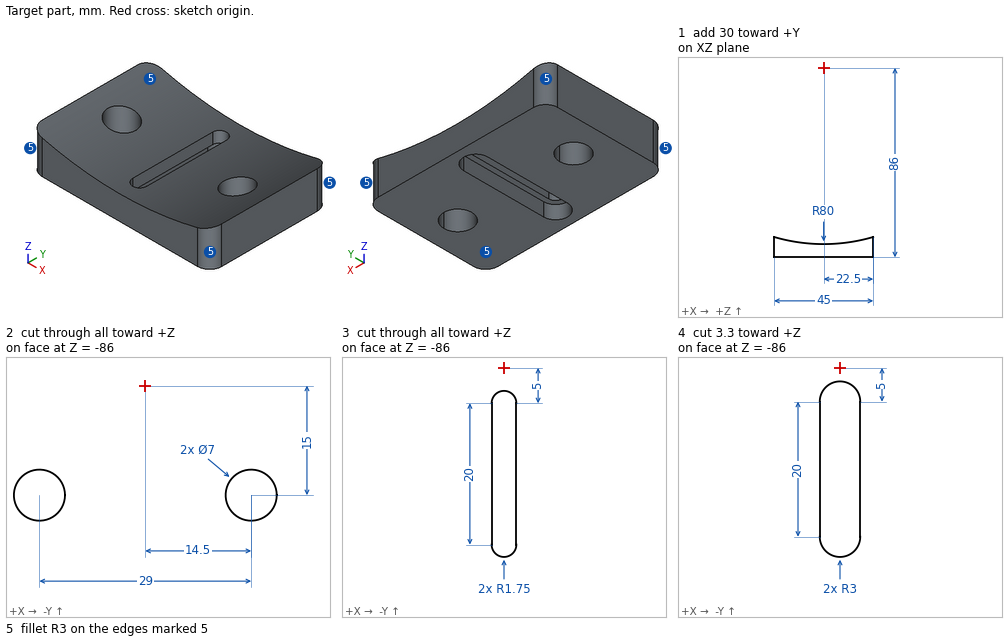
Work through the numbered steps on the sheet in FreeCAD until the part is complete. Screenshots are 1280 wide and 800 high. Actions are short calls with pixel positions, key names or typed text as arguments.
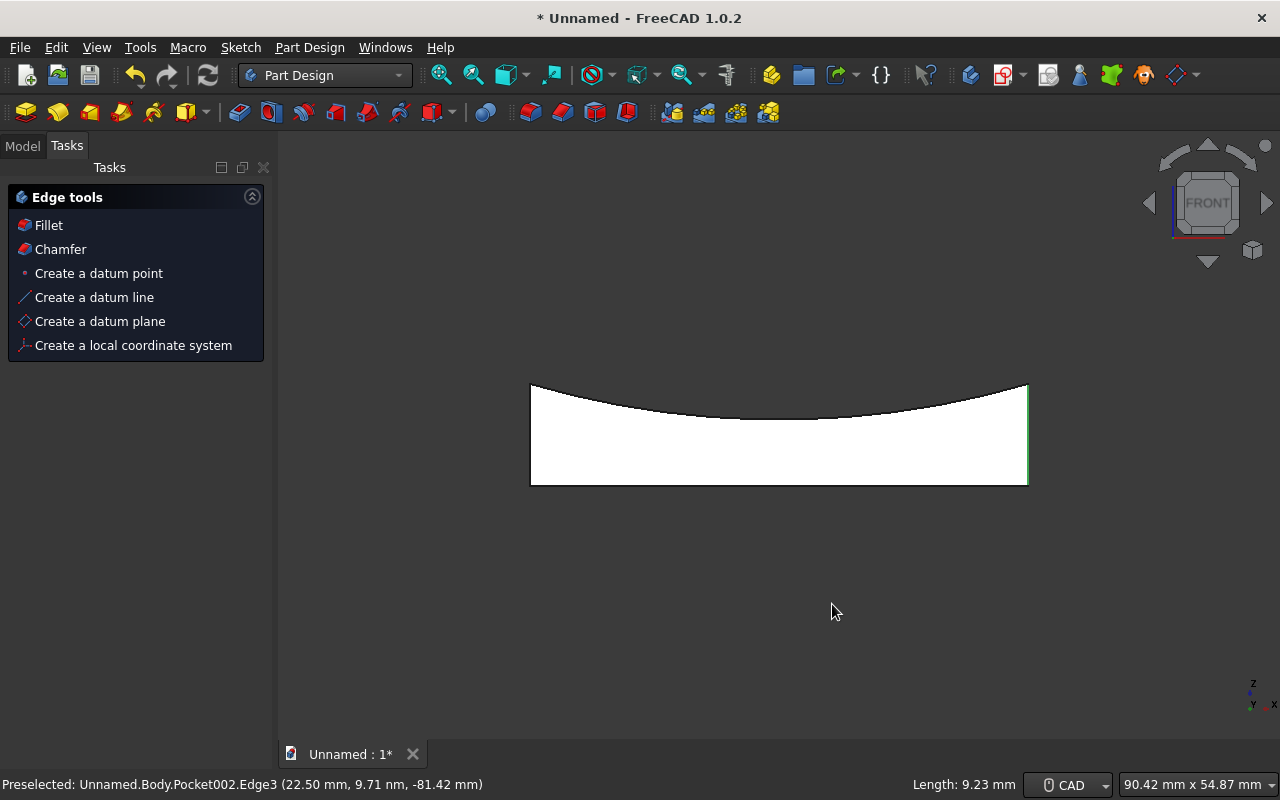
click(530, 473, ctrl)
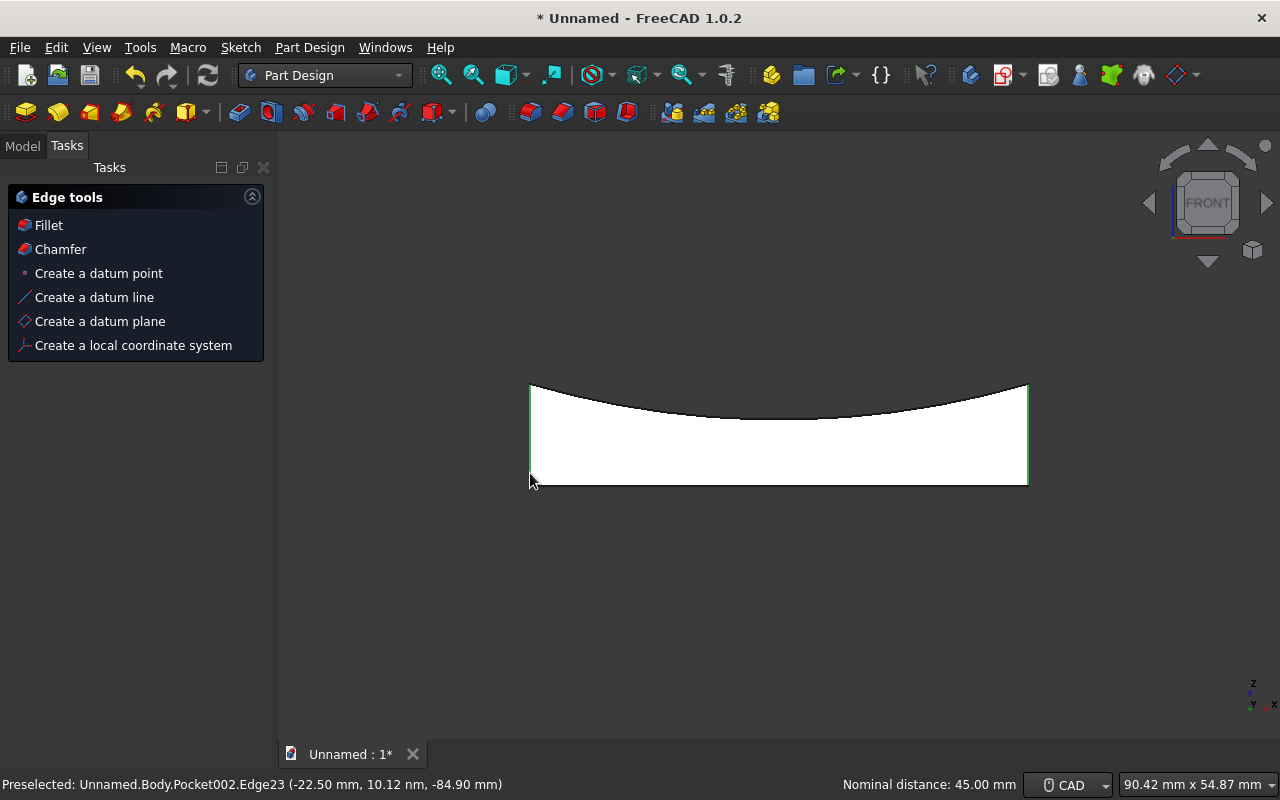
key(3)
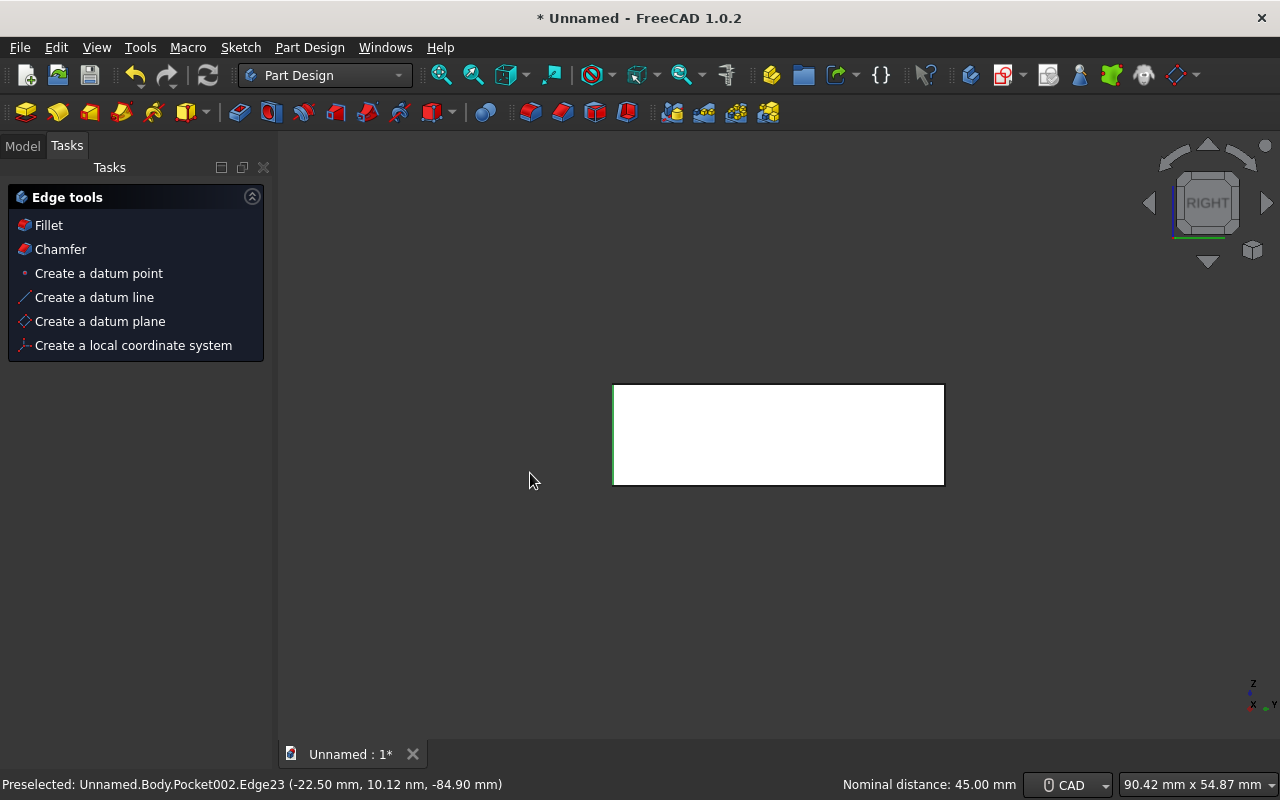
key(v)
key(f)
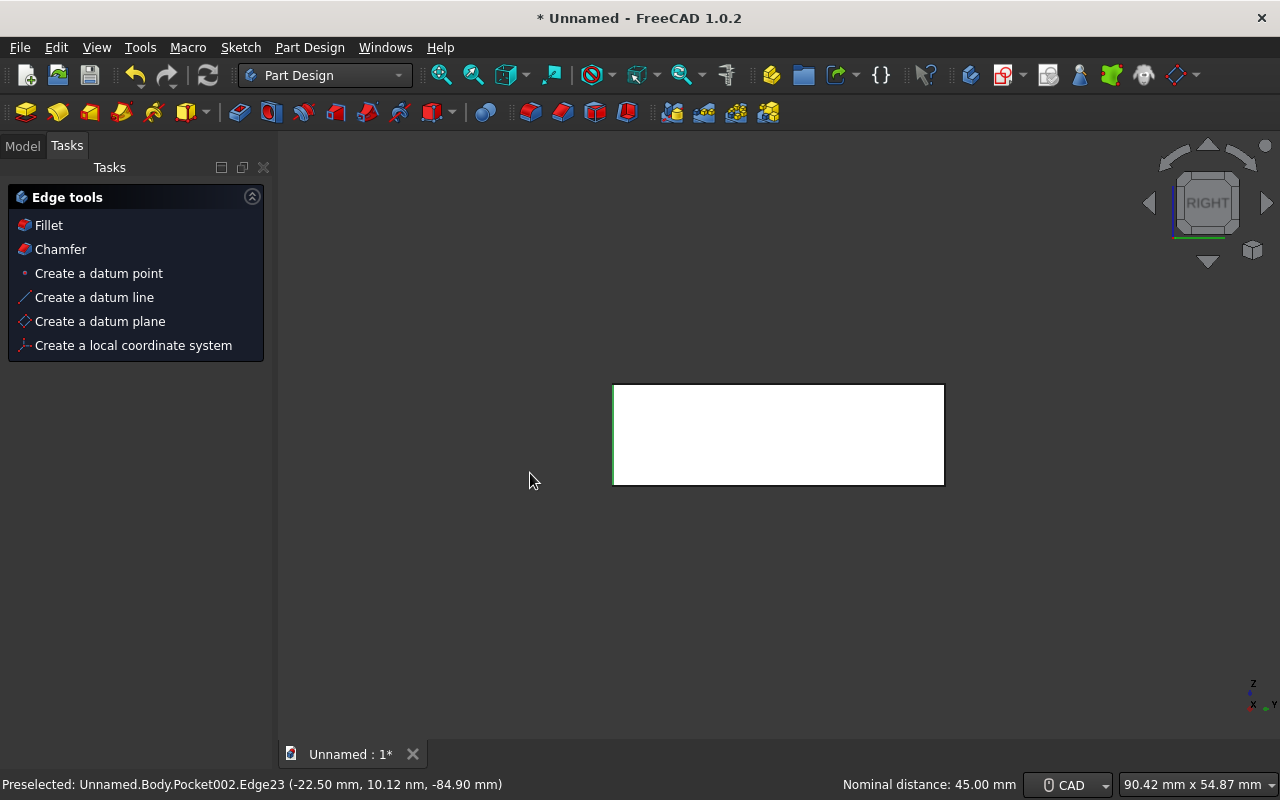
click(945, 434, ctrl)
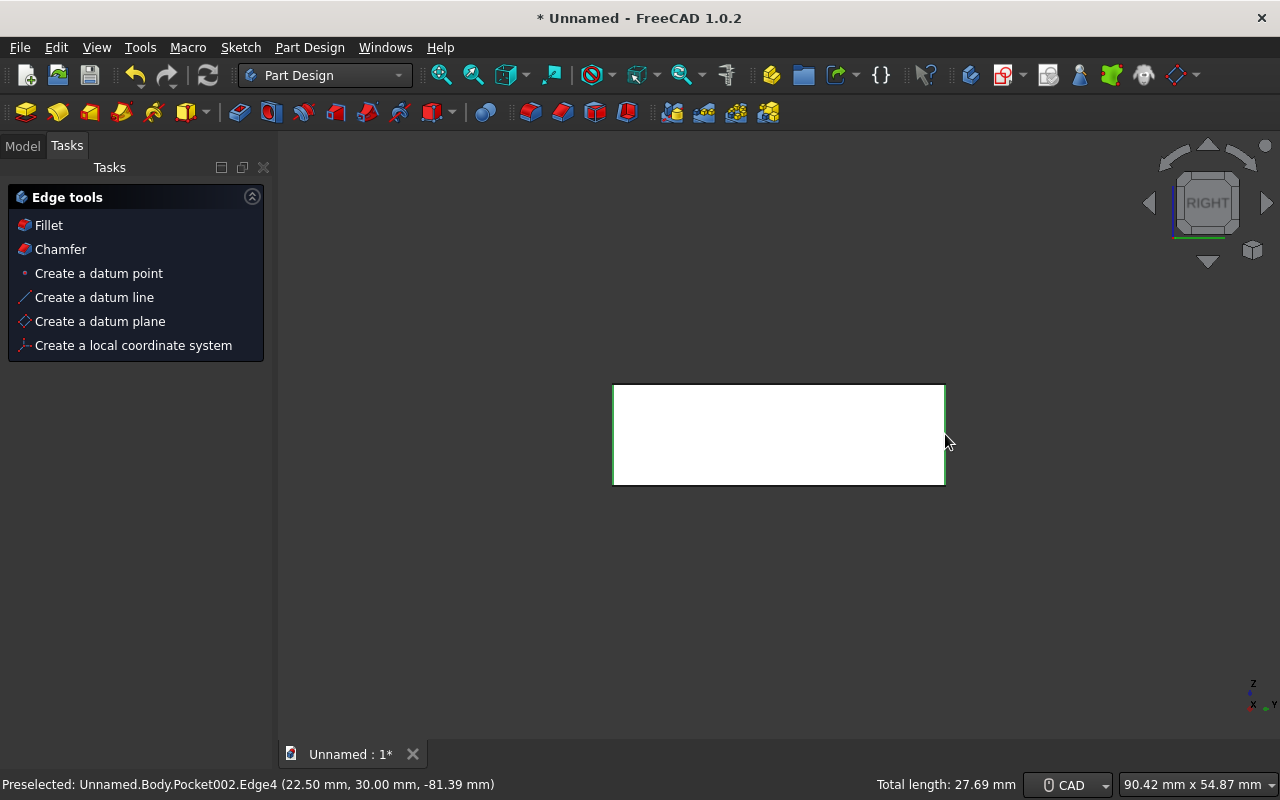
key(5)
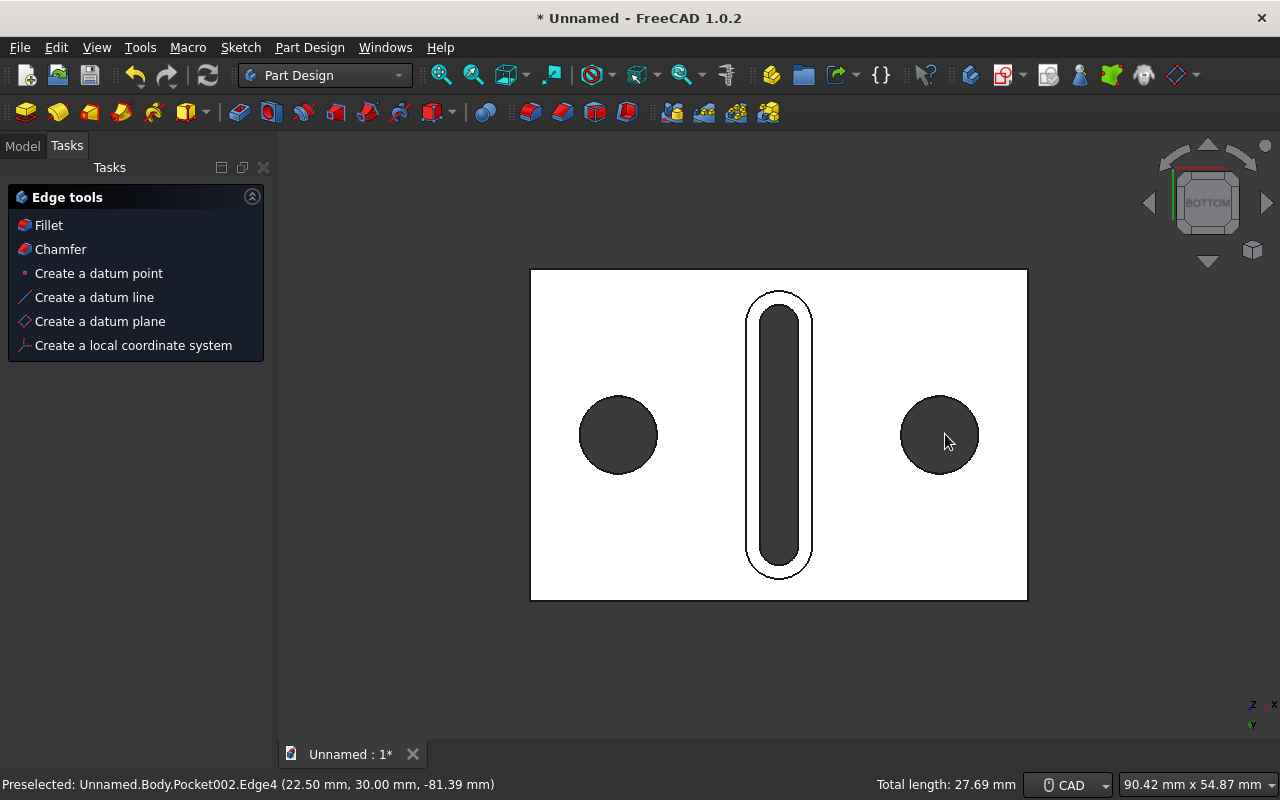
key(4)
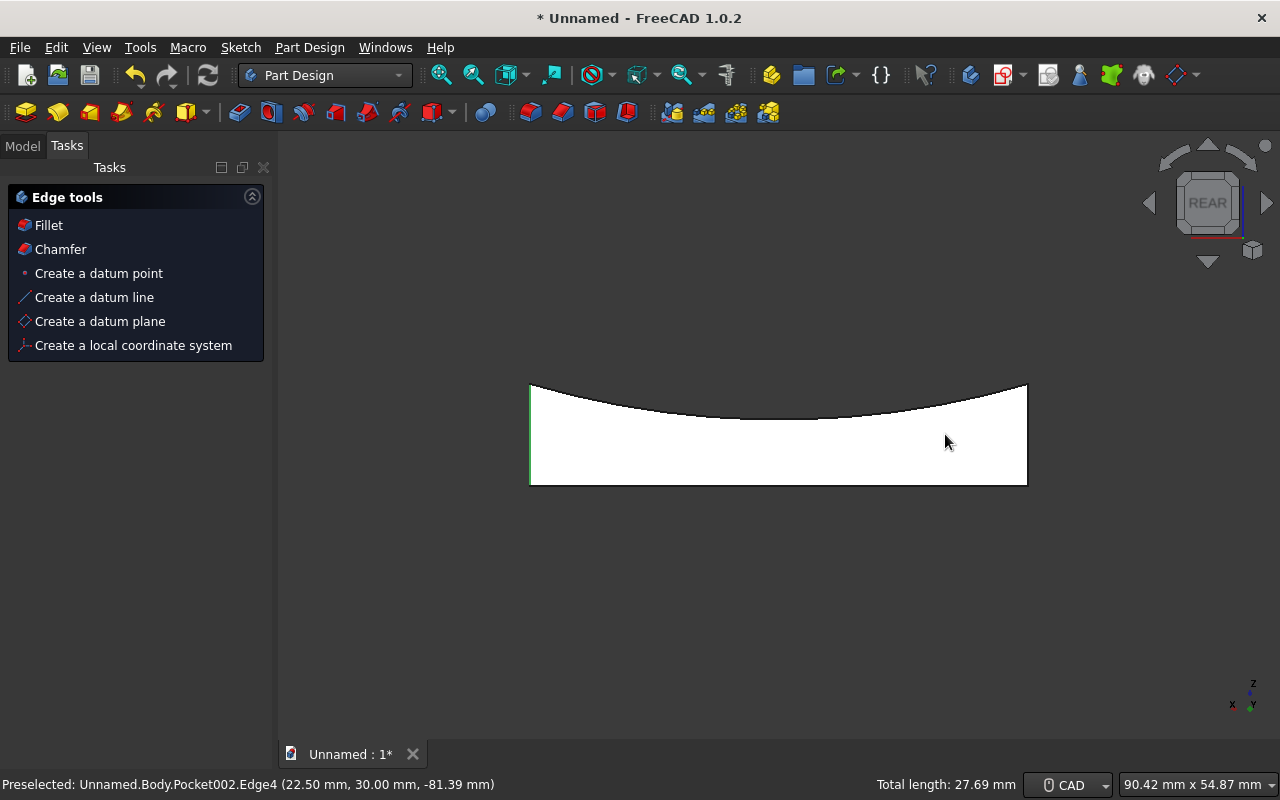
click(1028, 434, ctrl)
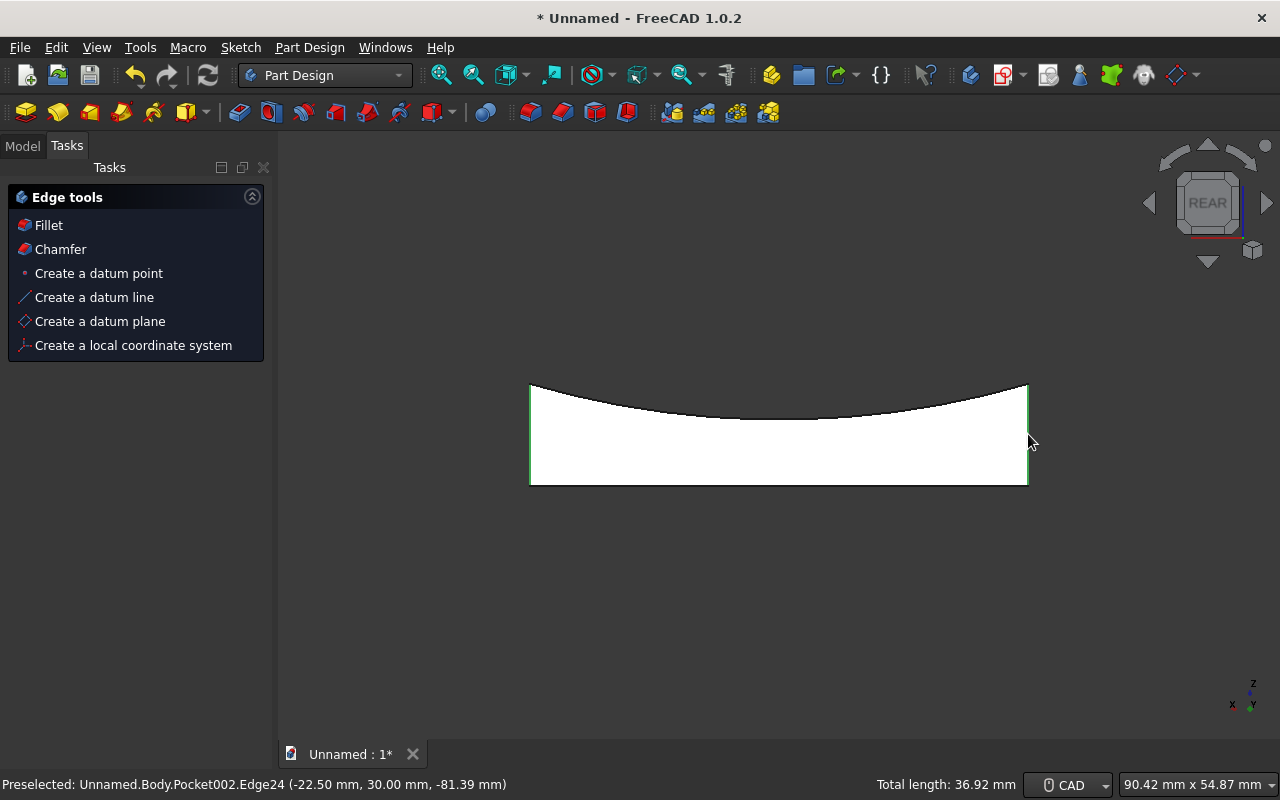
click(532, 112)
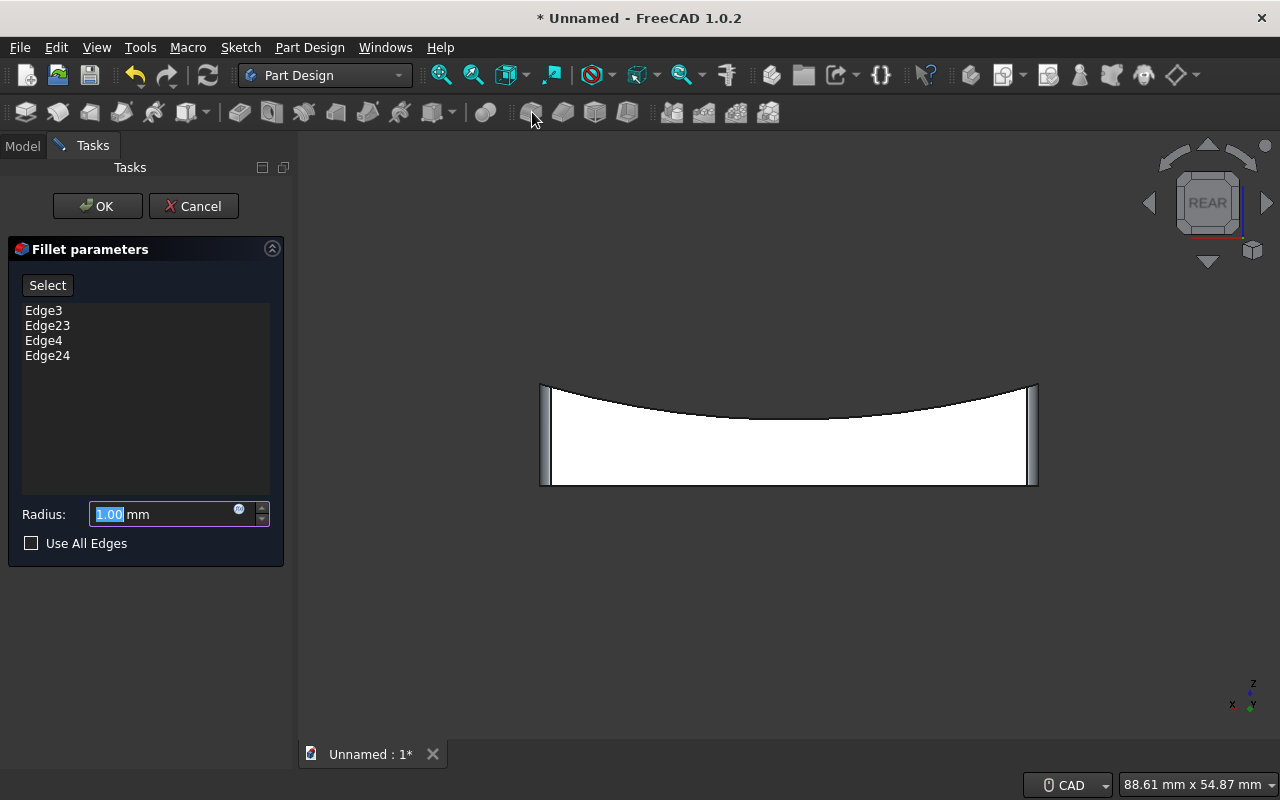
text(3)
key(Tab)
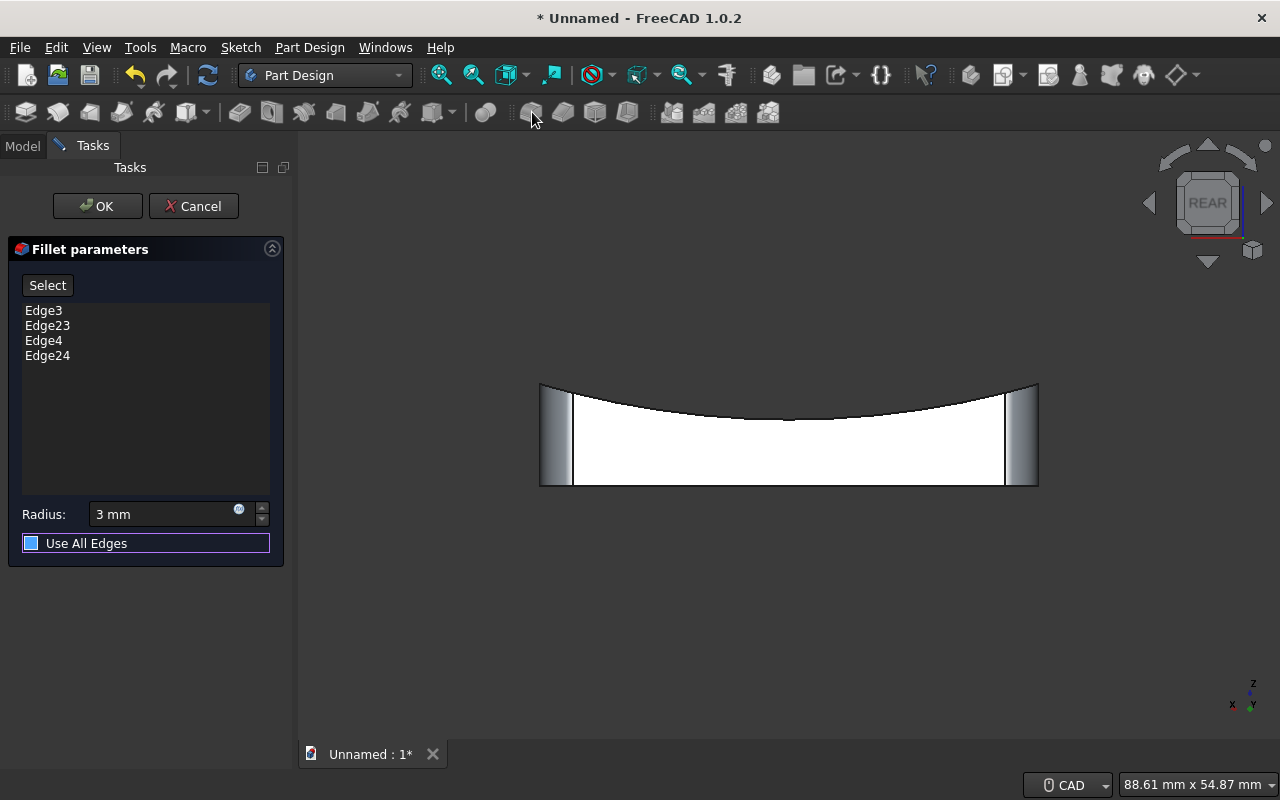
click(98, 206)